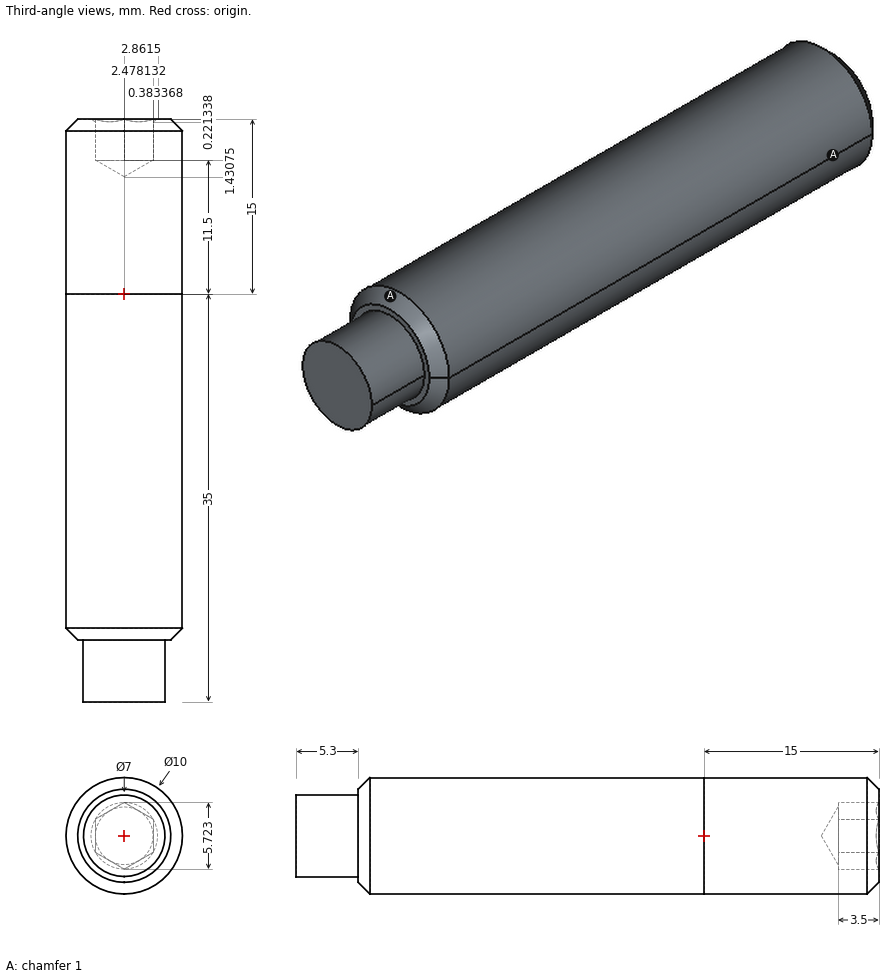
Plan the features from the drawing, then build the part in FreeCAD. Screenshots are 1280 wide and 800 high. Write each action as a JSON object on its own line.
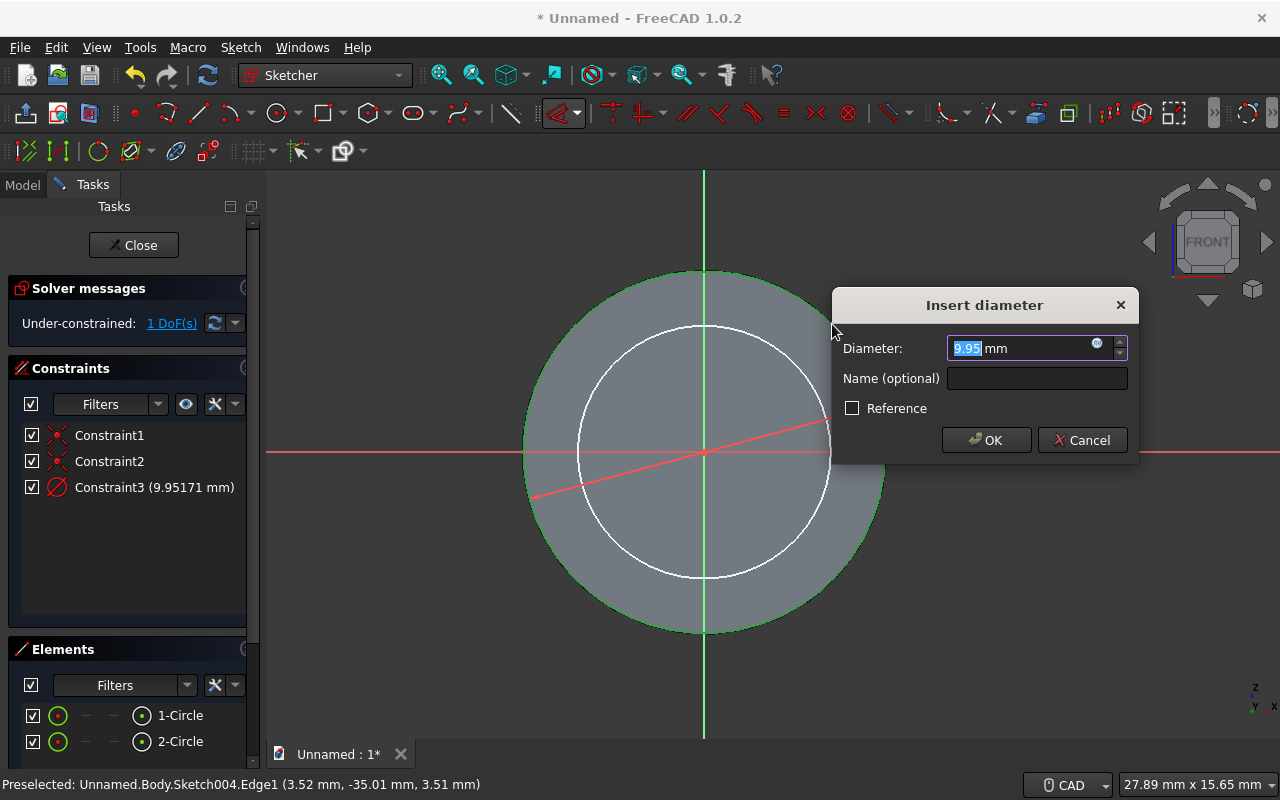
{"action": "type", "text": "10"}
{"action": "key", "text": "Return"}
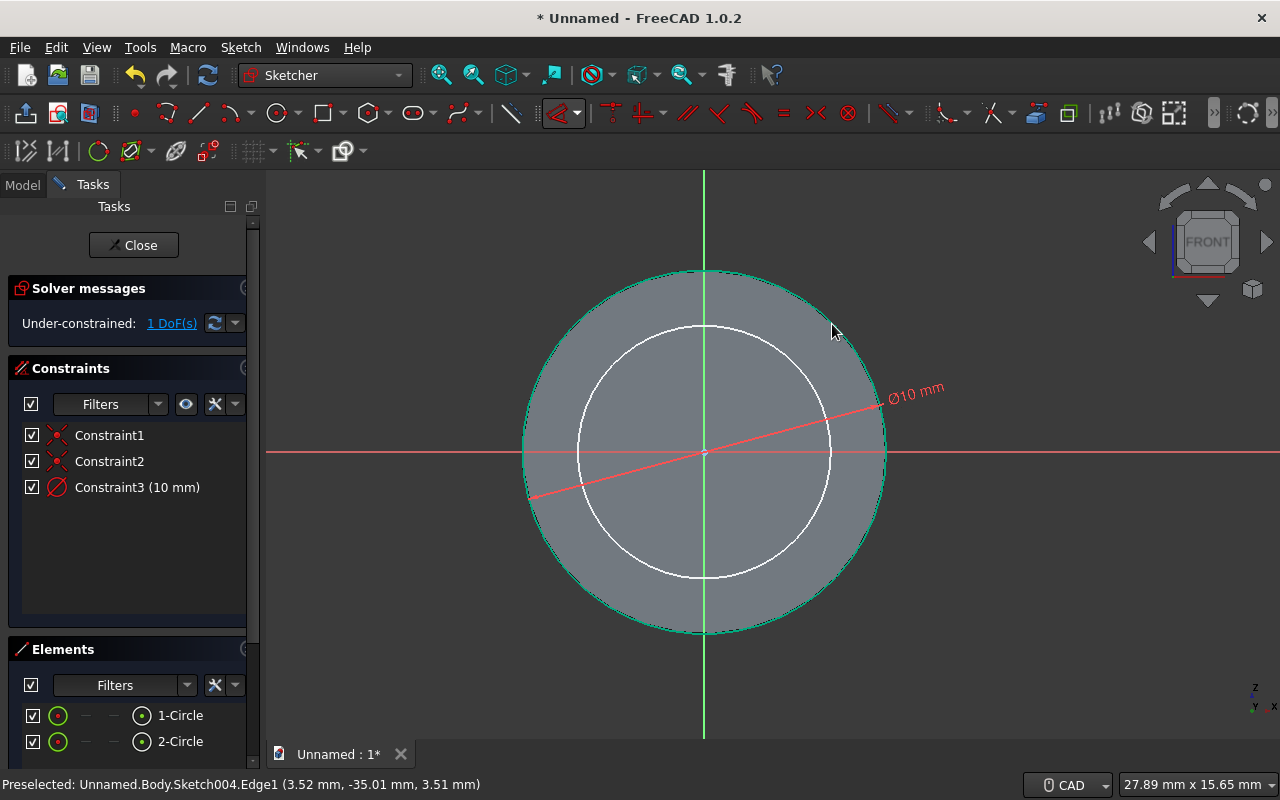
{"action": "left_click", "coordinate": [793, 362]}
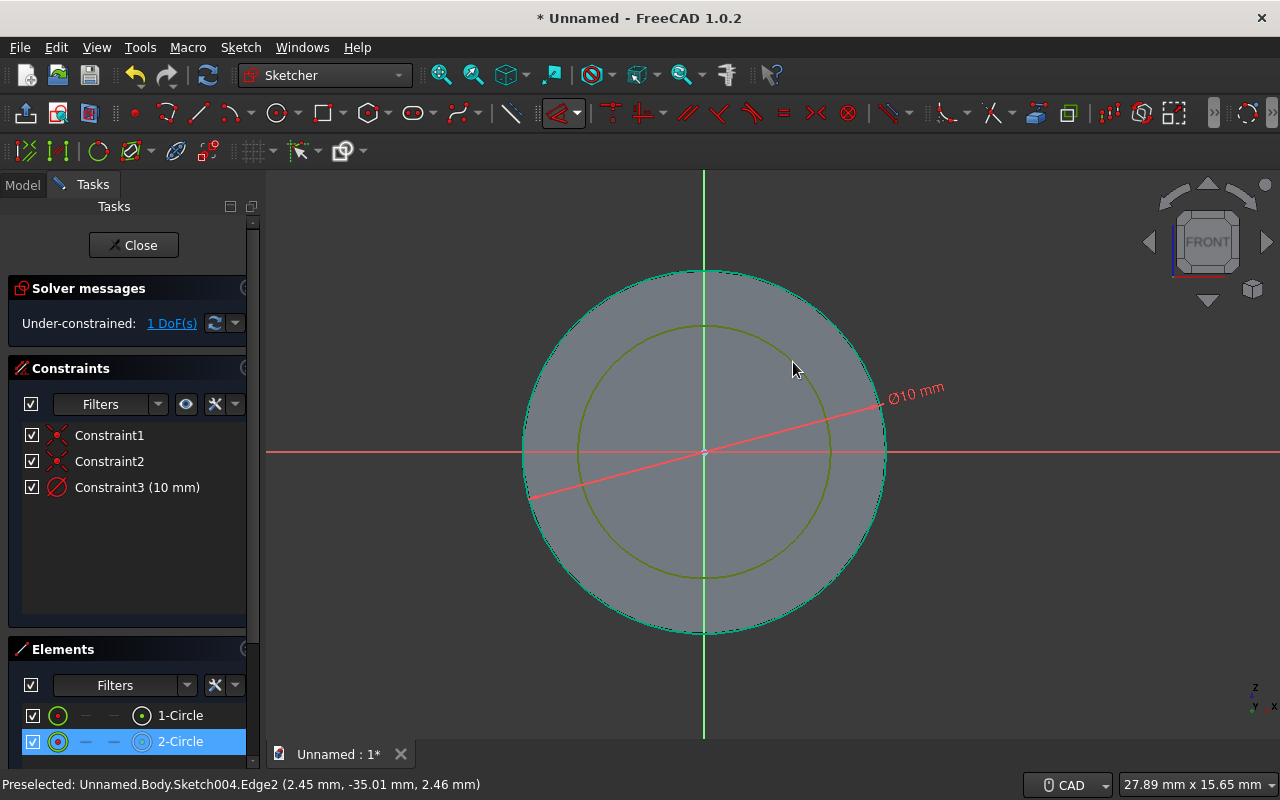
{"action": "left_click", "coordinate": [580, 114]}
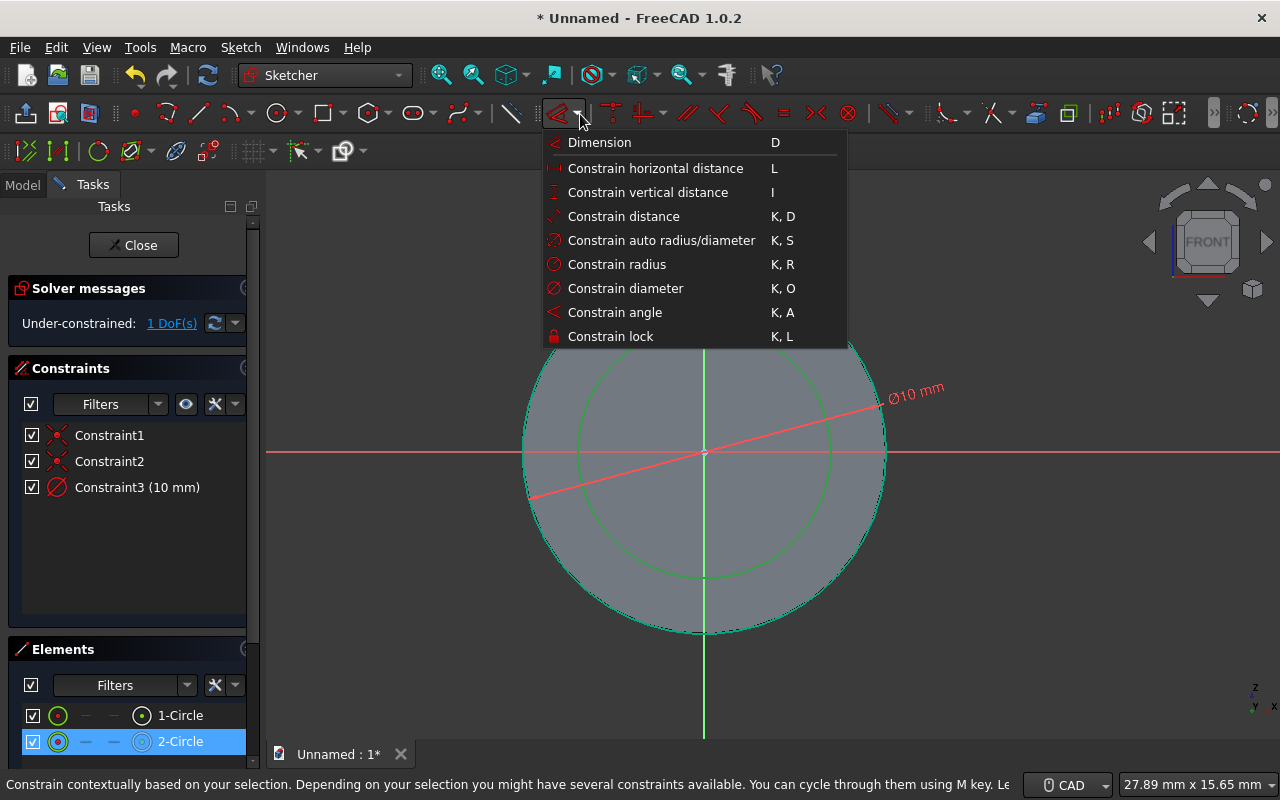
{"action": "left_click", "coordinate": [695, 288]}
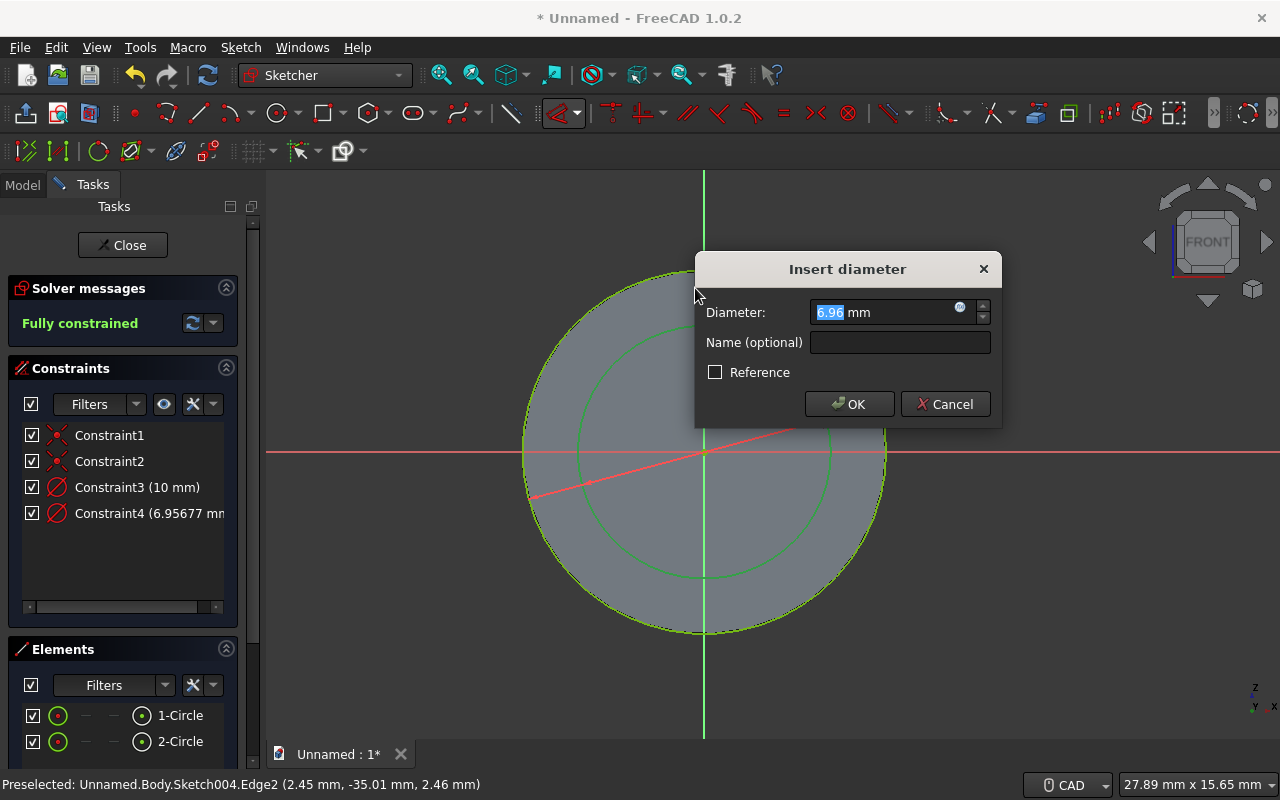
{"action": "type", "text": "7"}
{"action": "key", "text": "Return"}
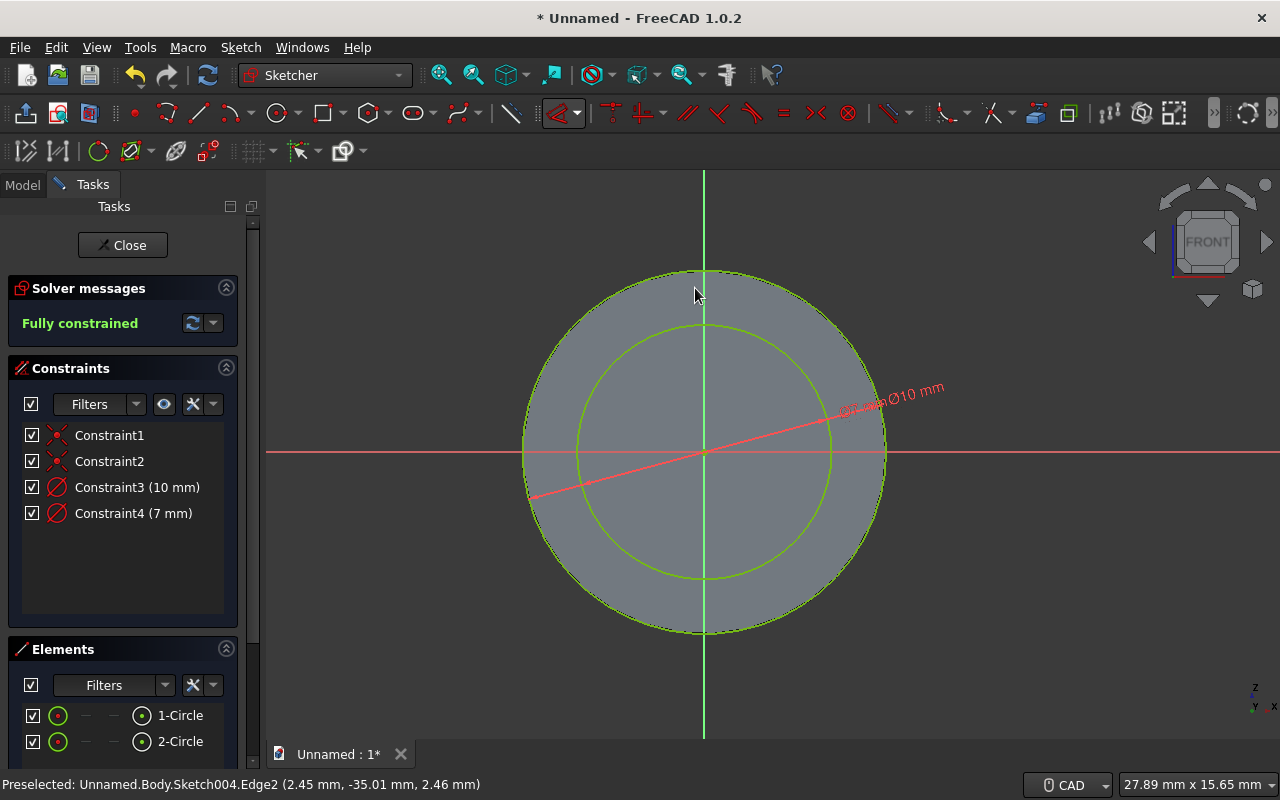
{"action": "left_click", "coordinate": [123, 245]}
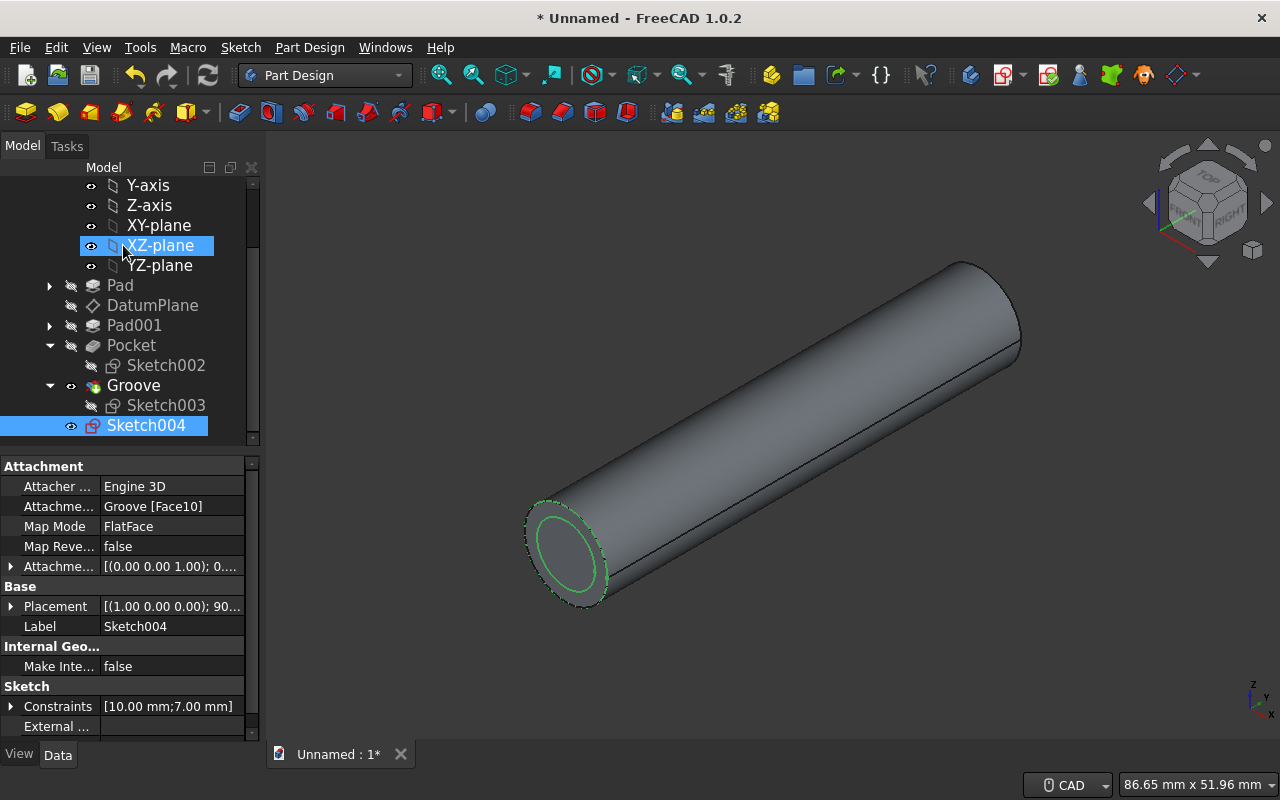
{"action": "left_click", "coordinate": [240, 112]}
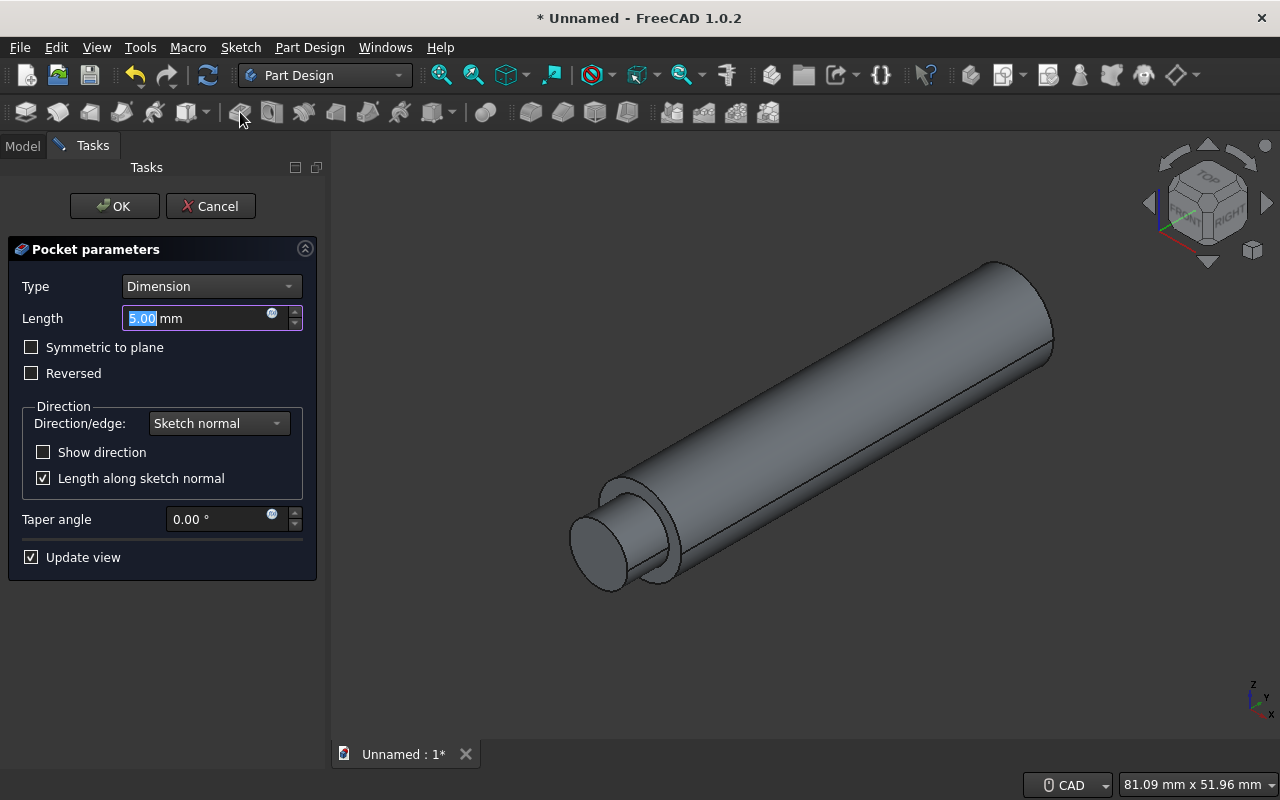
{"action": "type", "text": "5.3"}
{"action": "key", "text": "Tab"}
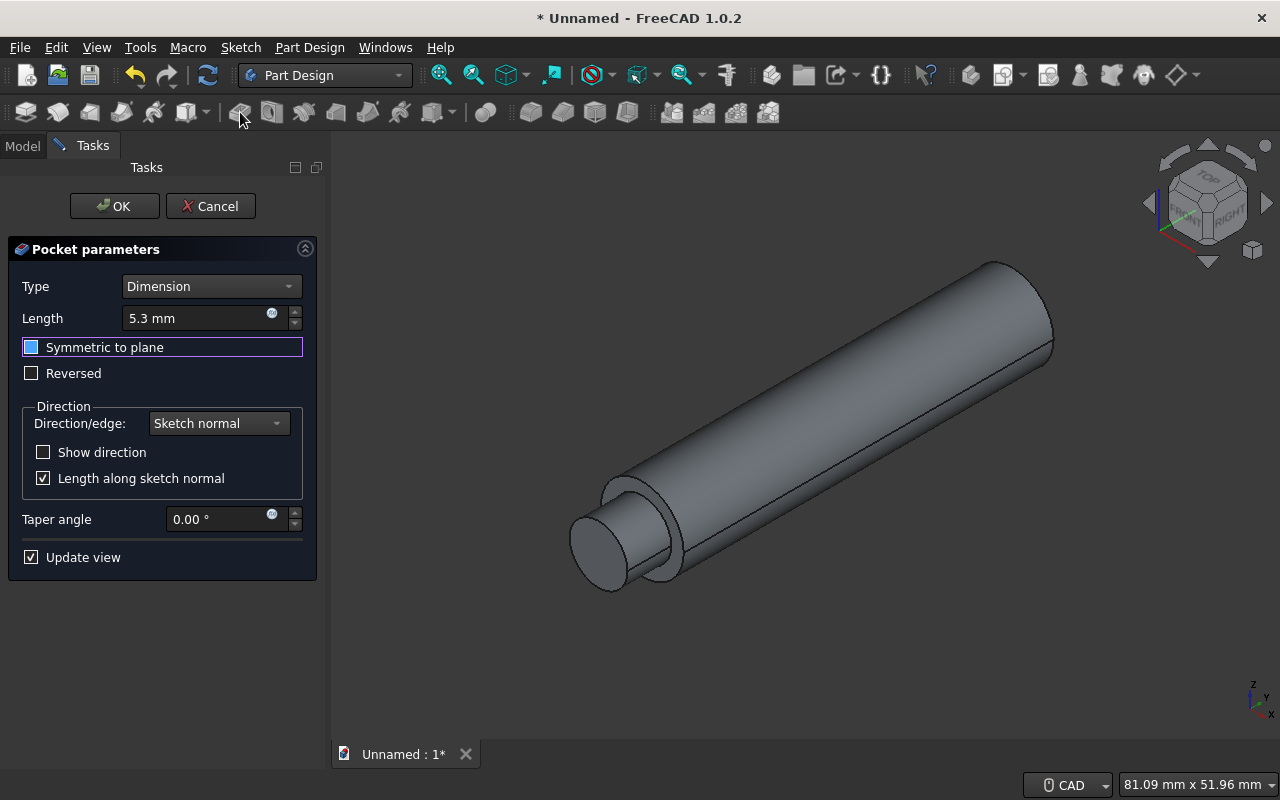
{"action": "left_click", "coordinate": [115, 206]}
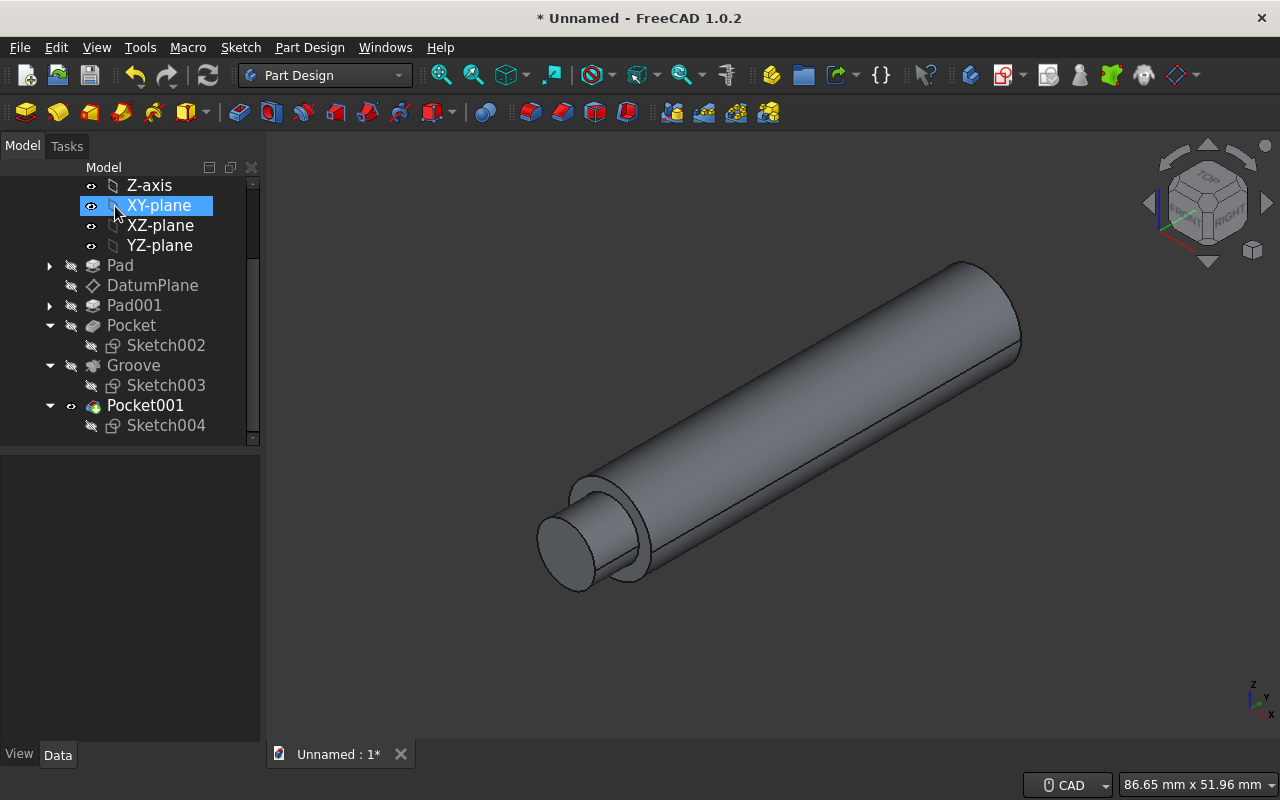
{"action": "left_click", "coordinate": [576, 481]}